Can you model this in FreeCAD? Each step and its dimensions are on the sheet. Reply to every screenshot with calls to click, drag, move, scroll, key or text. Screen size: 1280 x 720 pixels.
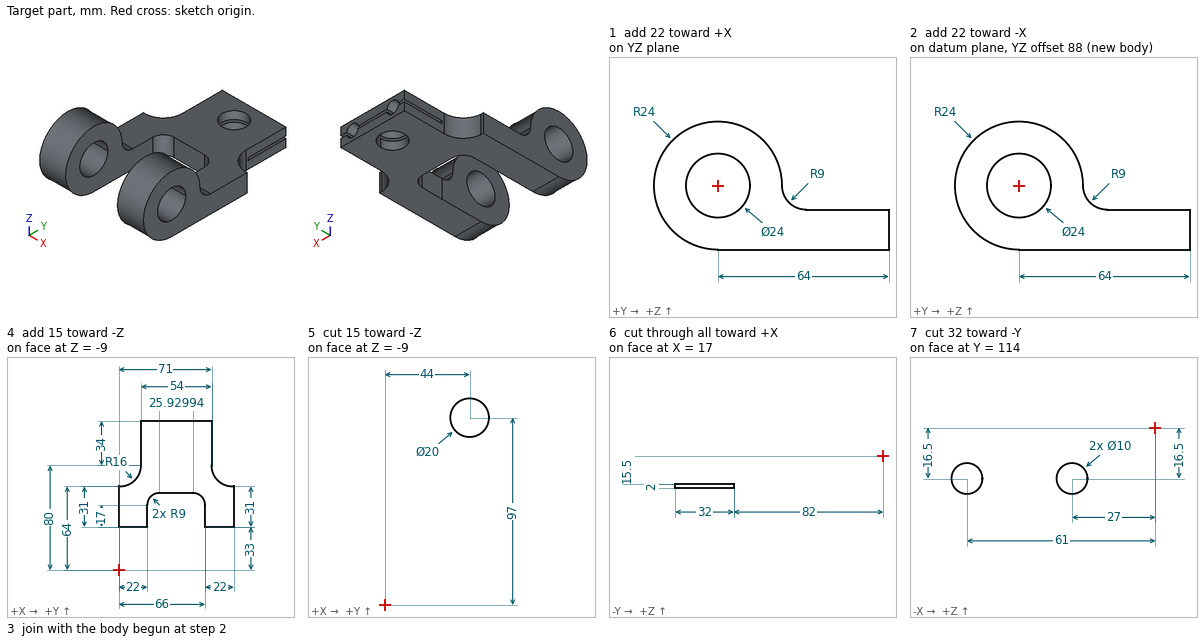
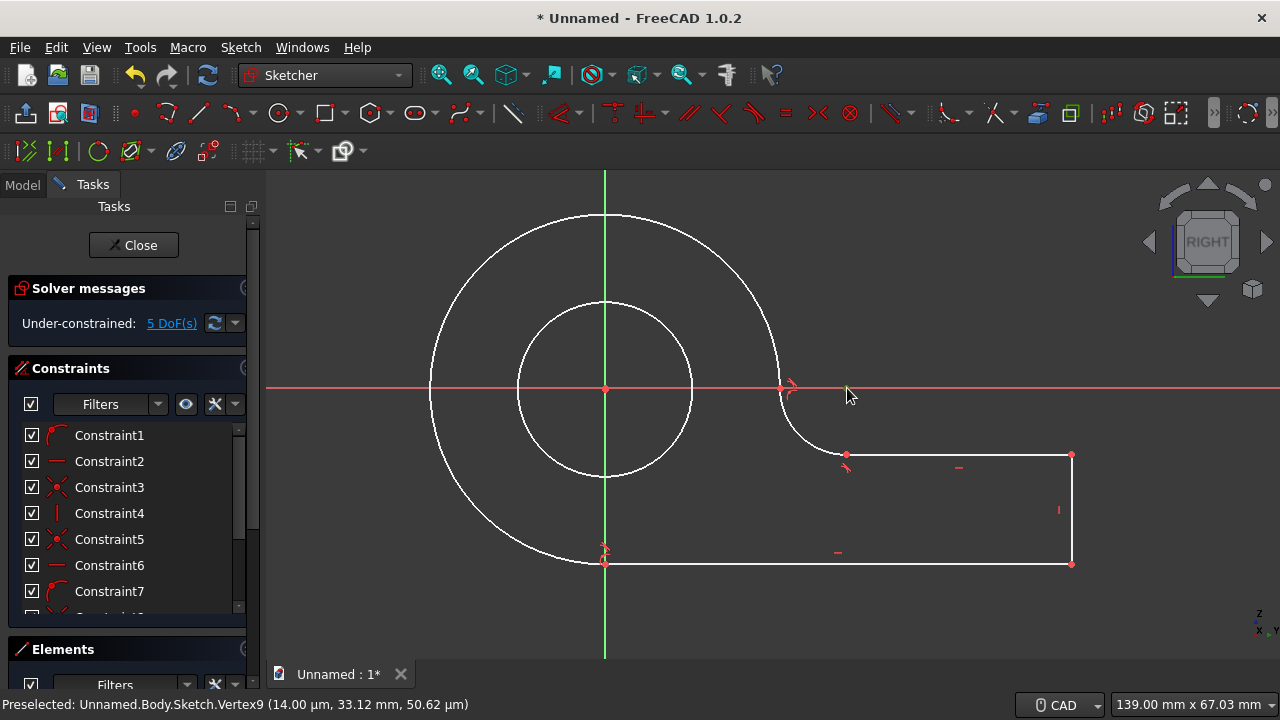
click(353, 388)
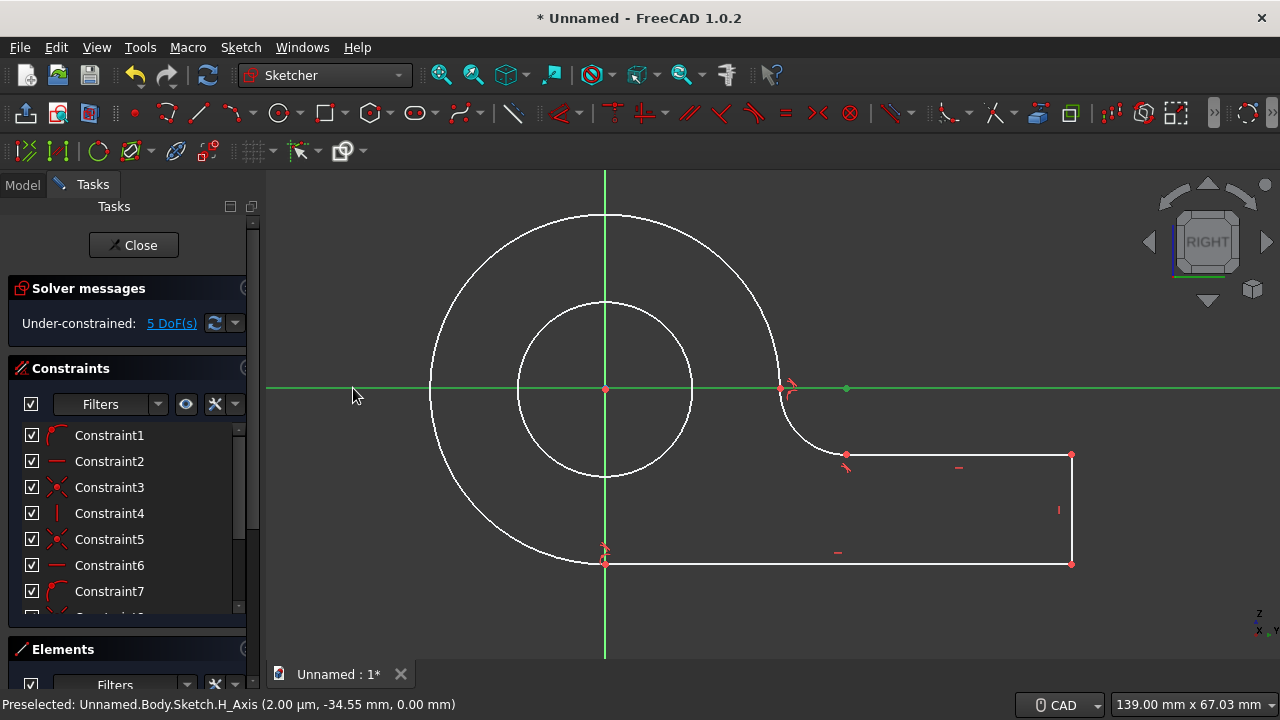
click(614, 114)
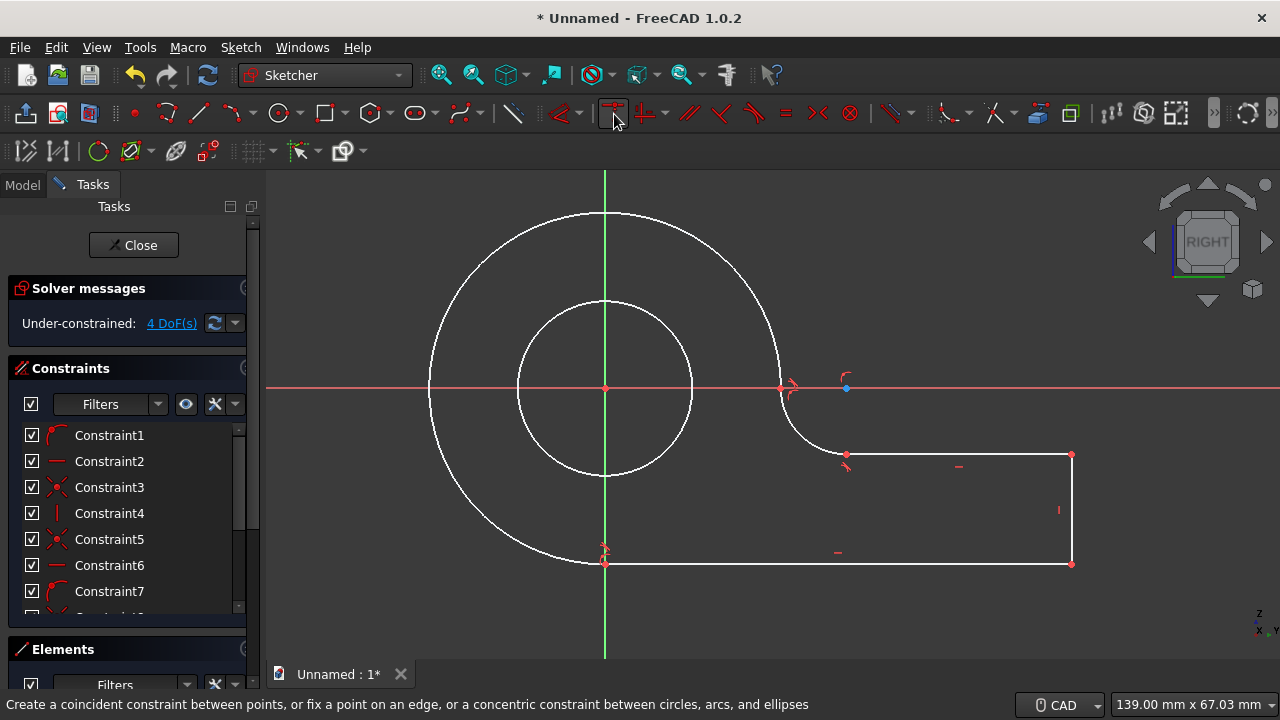
click(788, 418)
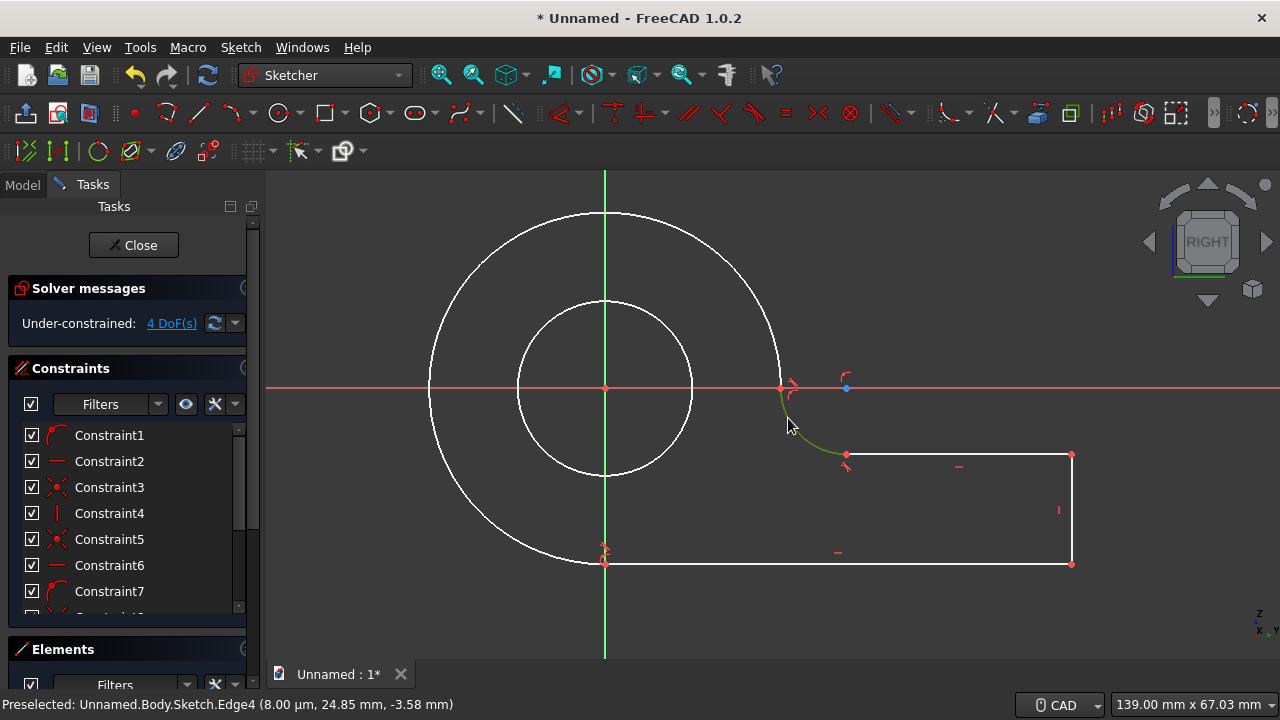
click(582, 114)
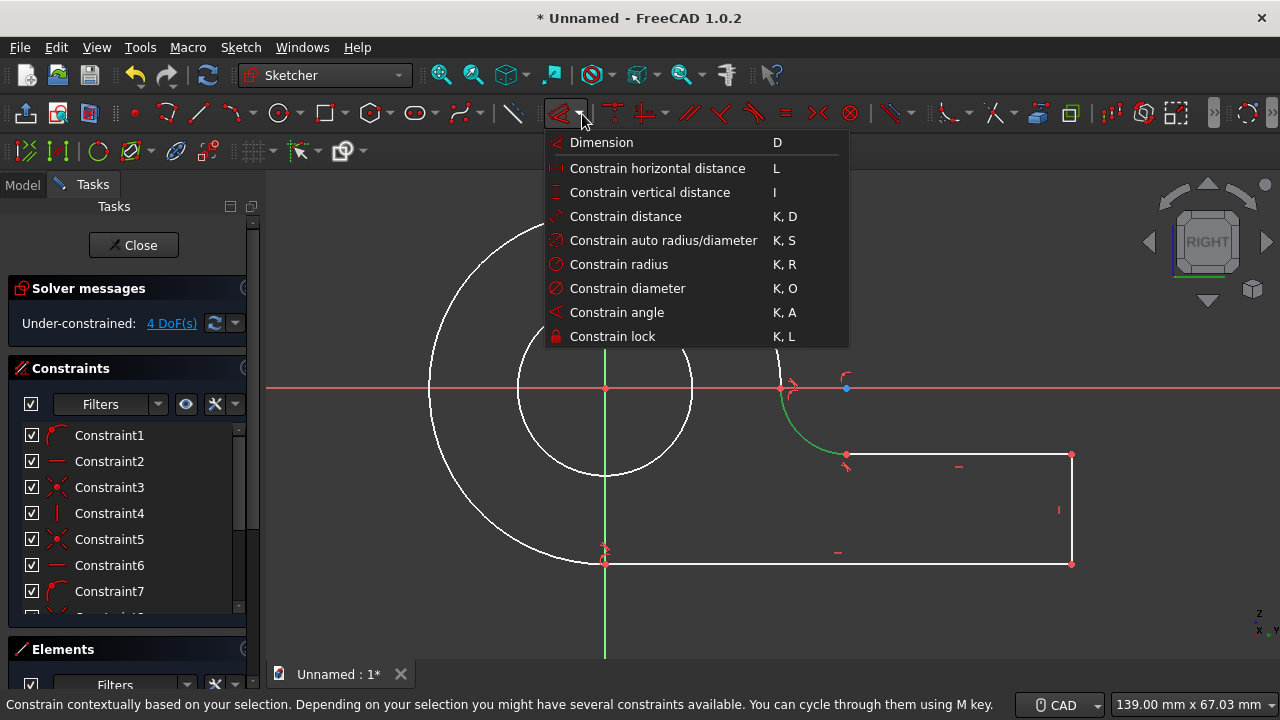
click(697, 264)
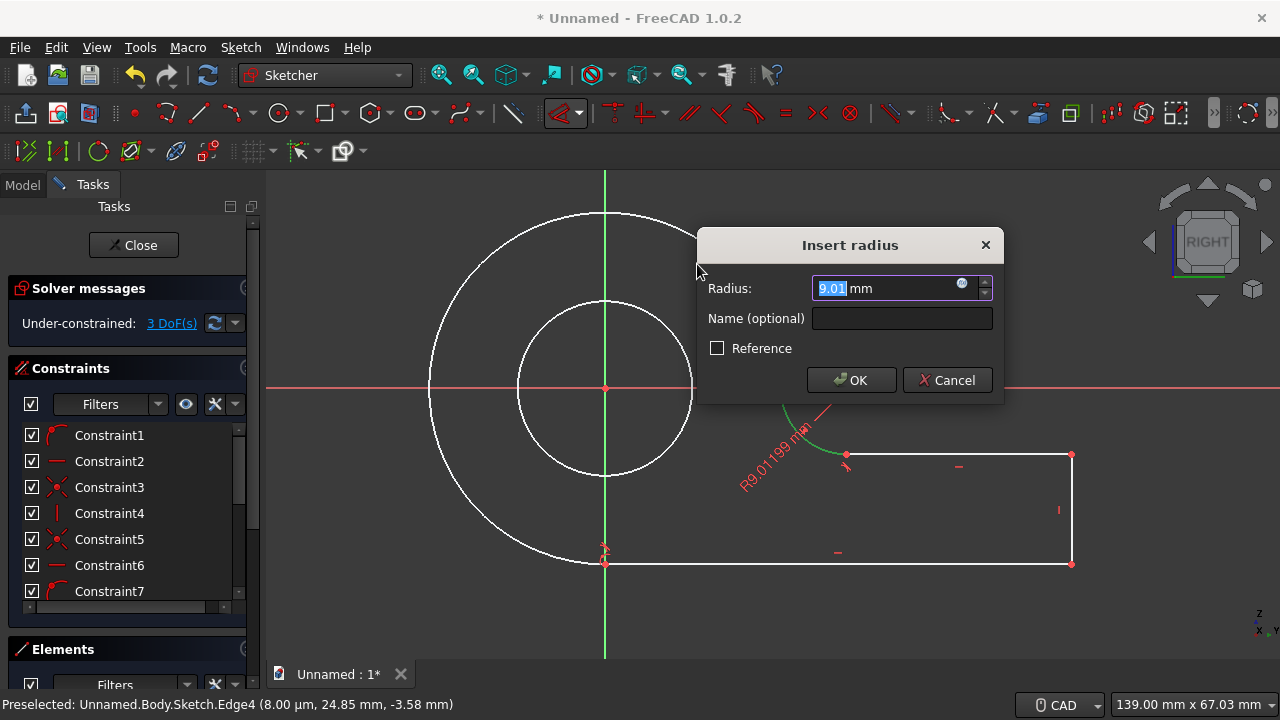
text(9)
key(Return)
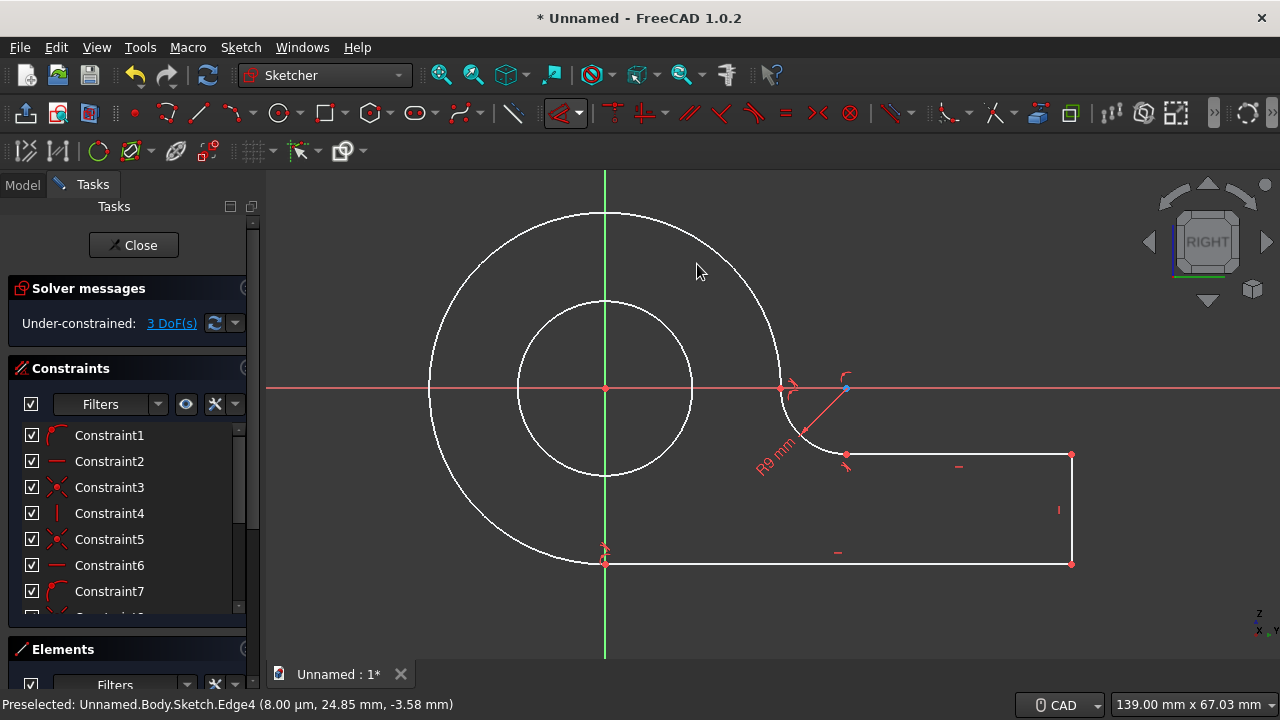
click(633, 215)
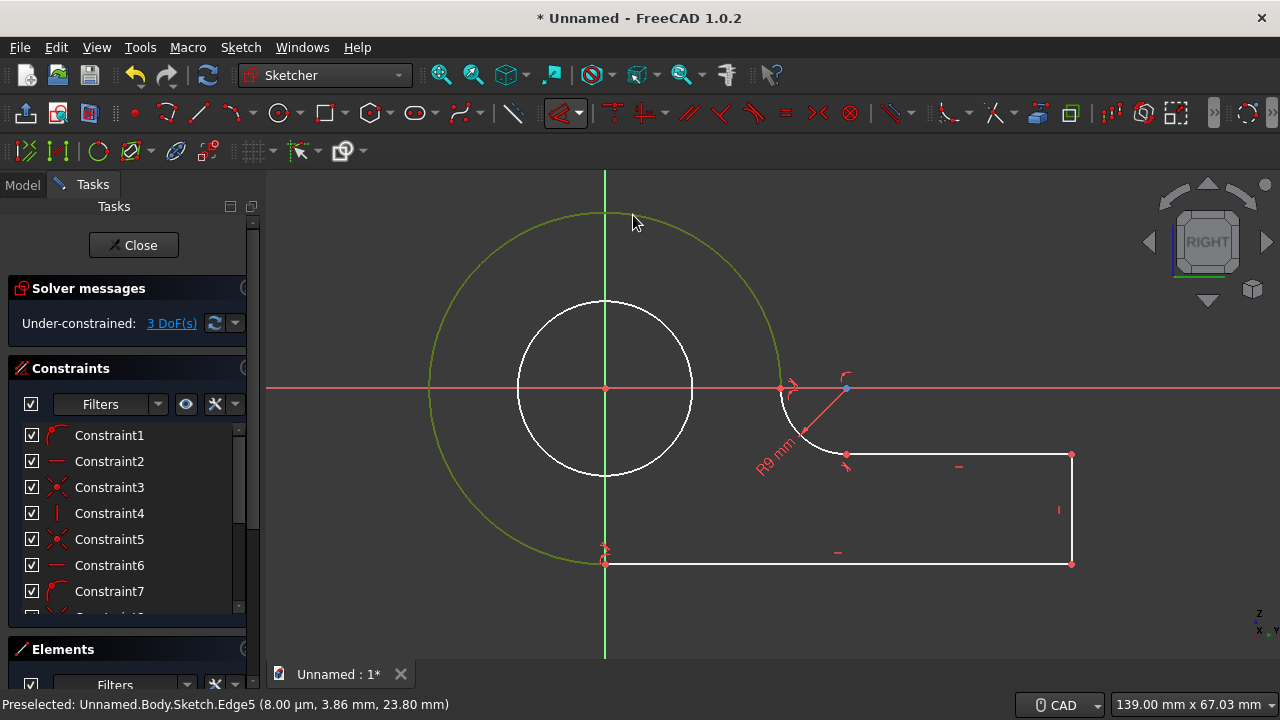
click(582, 114)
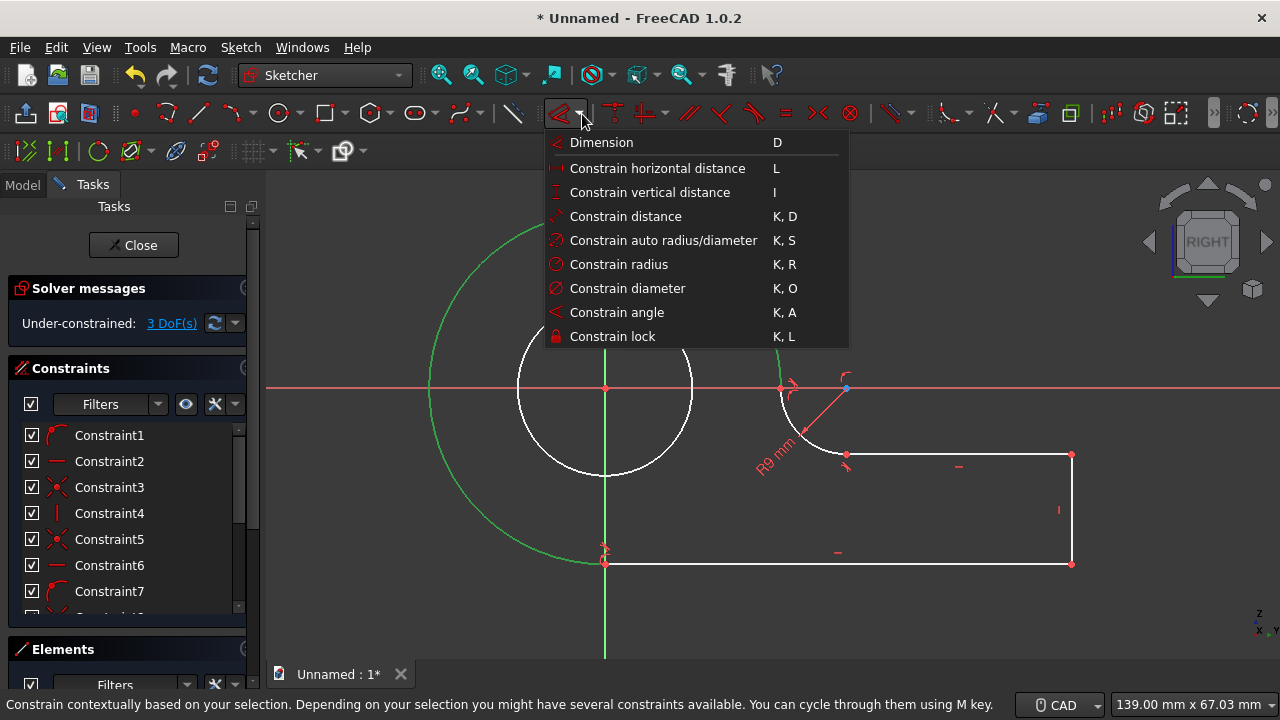
click(697, 264)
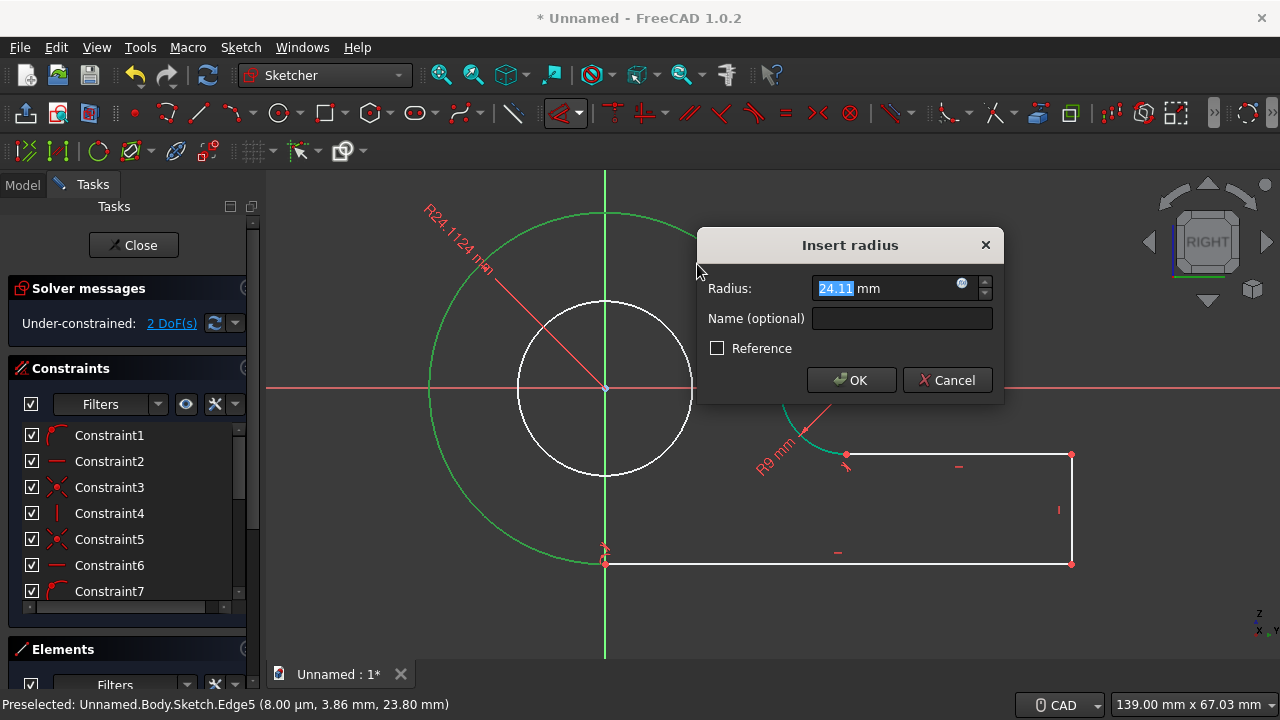
text(24)
key(Return)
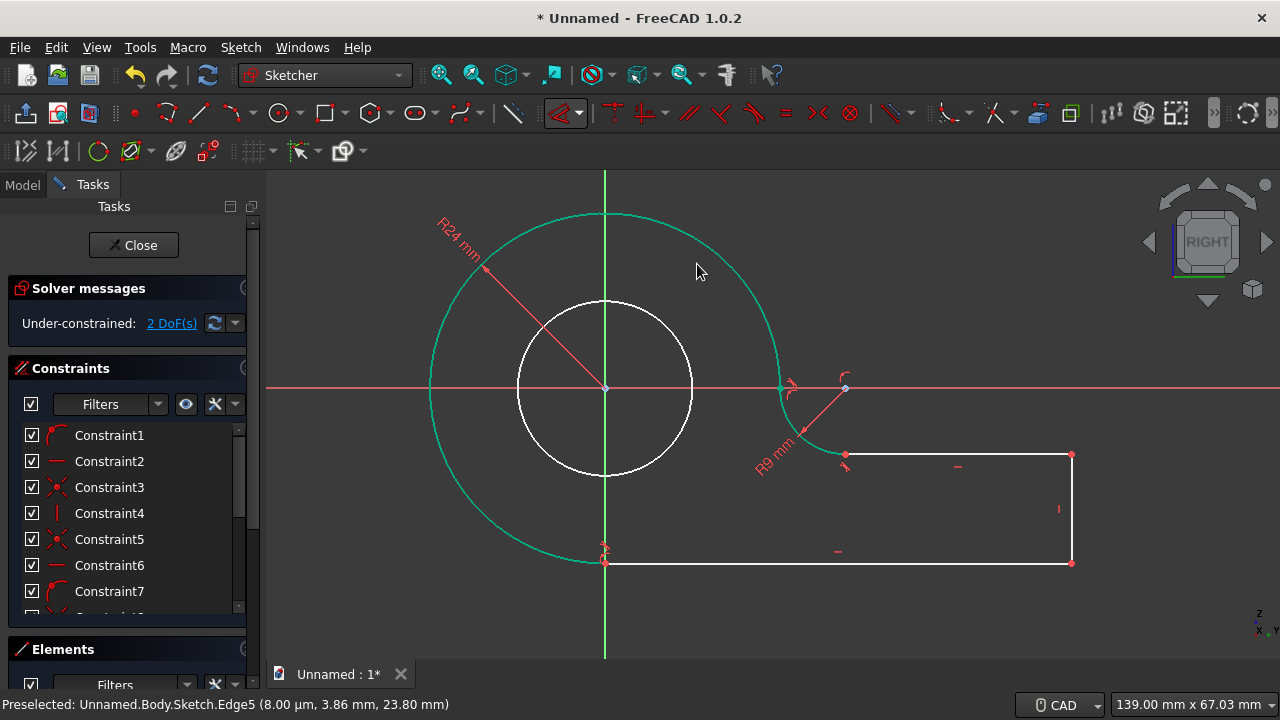
click(667, 327)